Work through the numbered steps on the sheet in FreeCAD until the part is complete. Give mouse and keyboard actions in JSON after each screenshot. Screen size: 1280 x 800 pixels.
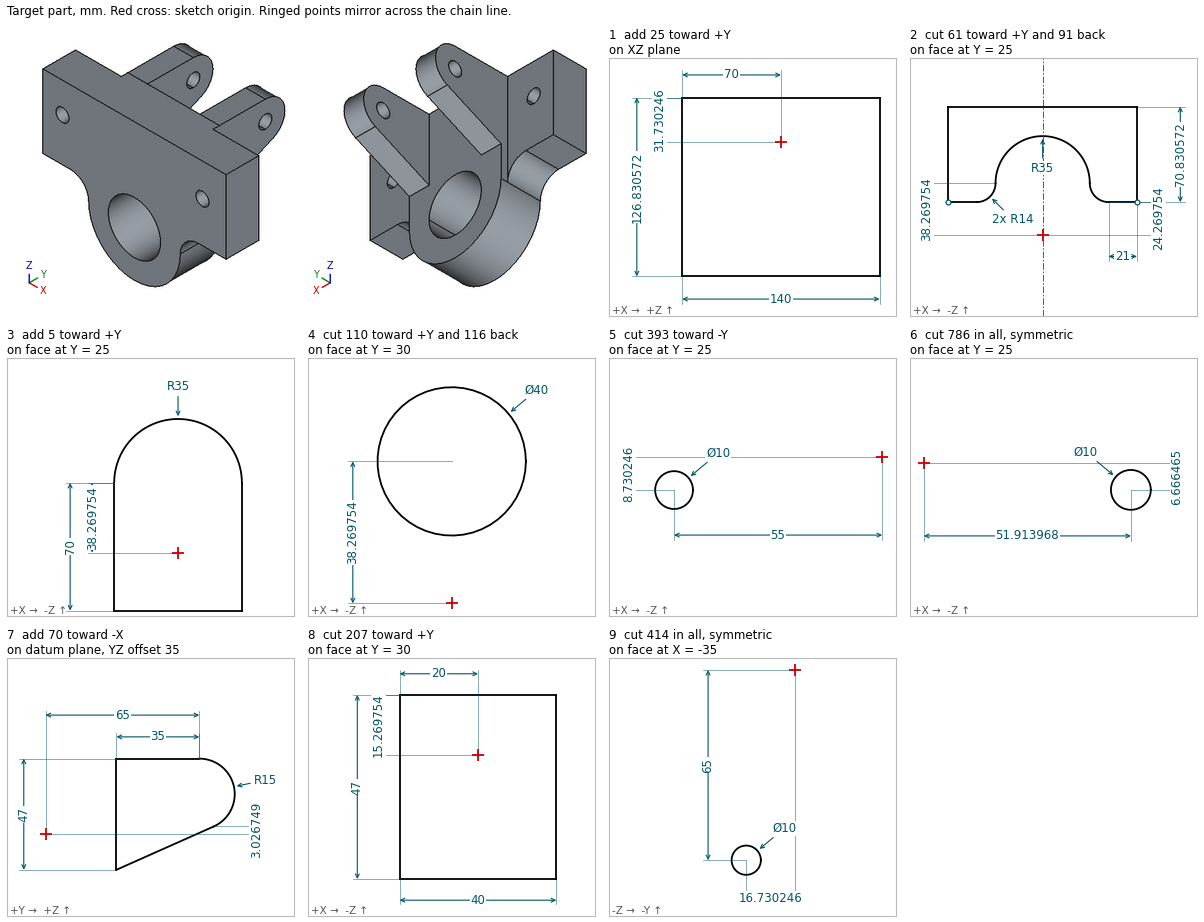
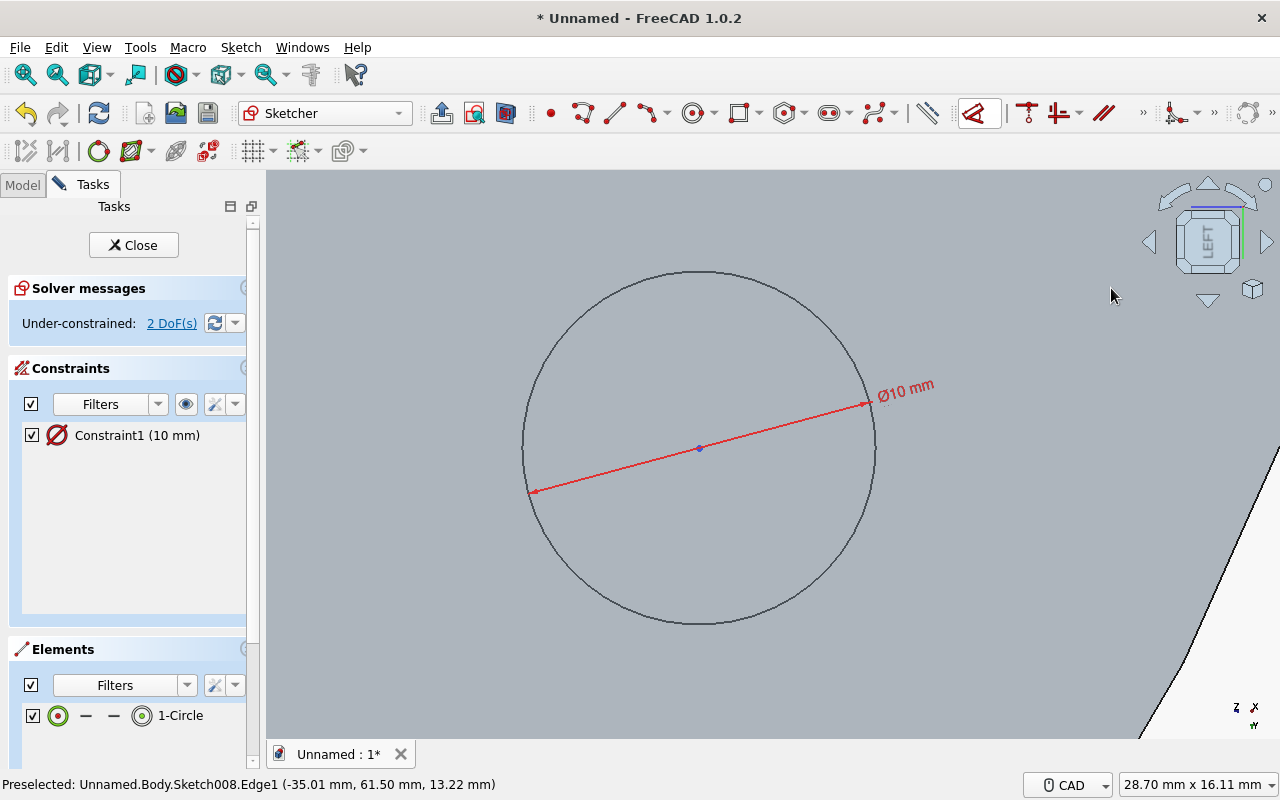
{"action": "left_click", "coordinate": [699, 448]}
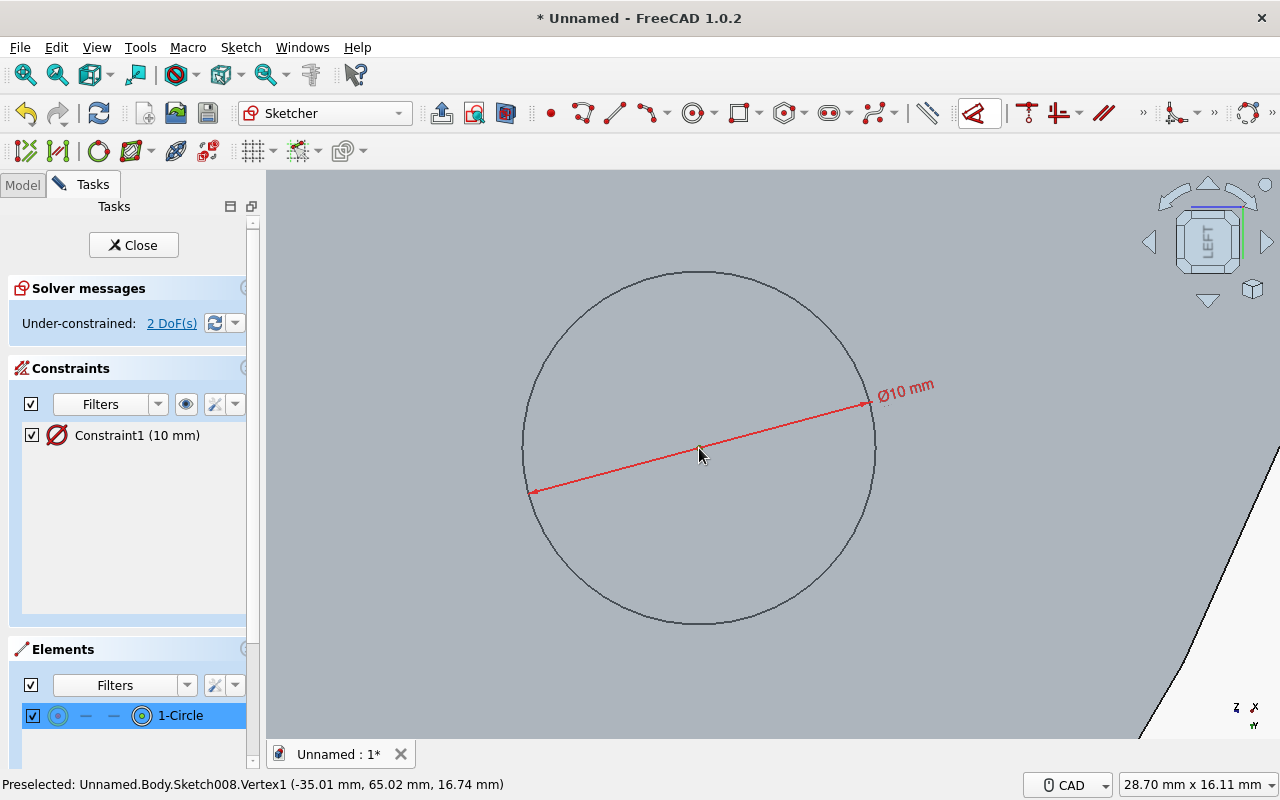
{"action": "key", "text": "i"}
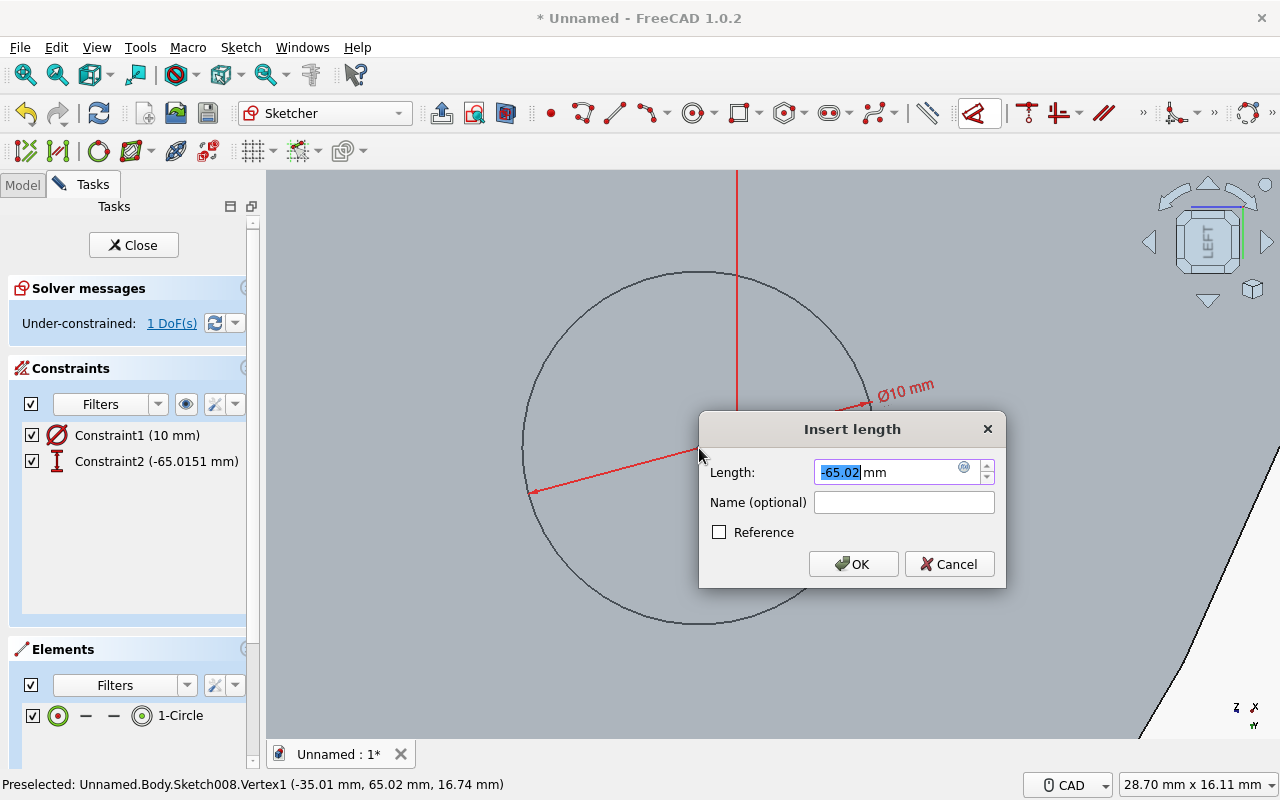
{"action": "type", "text": "-65"}
{"action": "key", "text": "Return"}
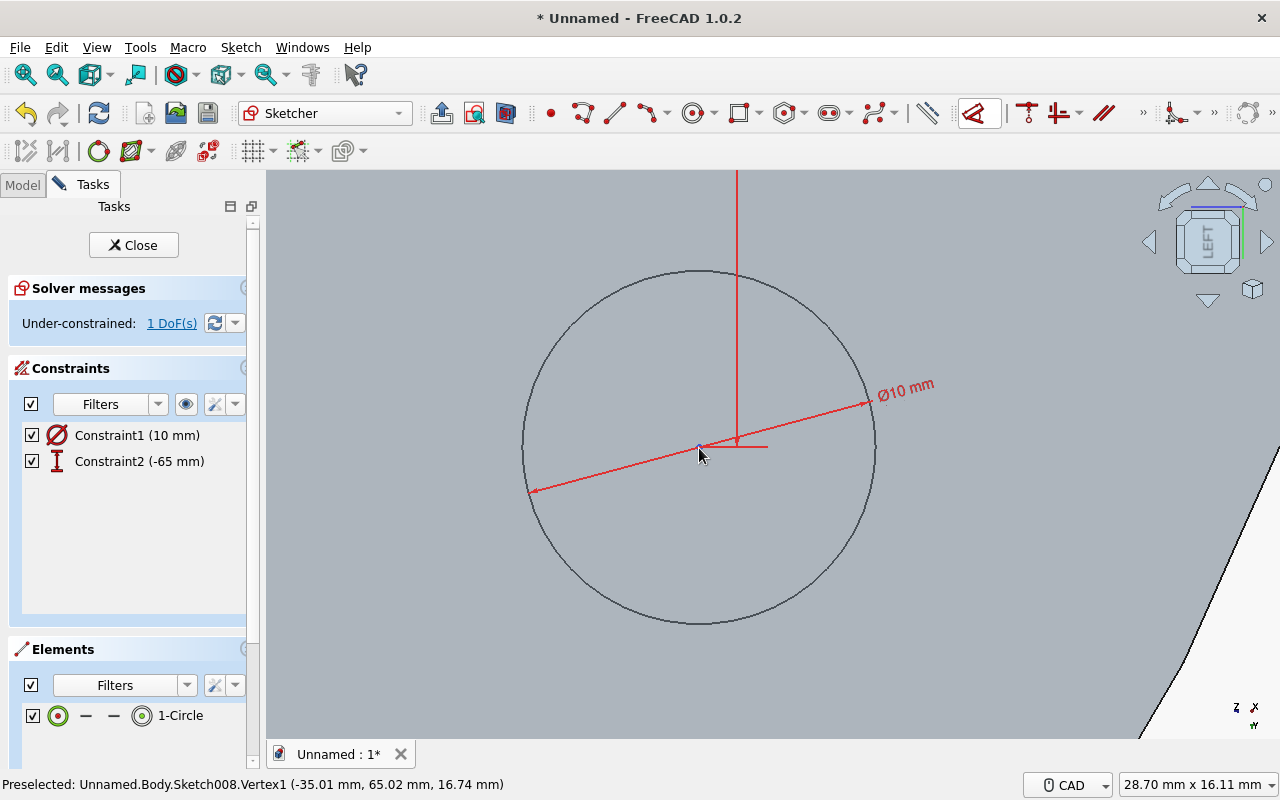
{"action": "left_click", "coordinate": [699, 447]}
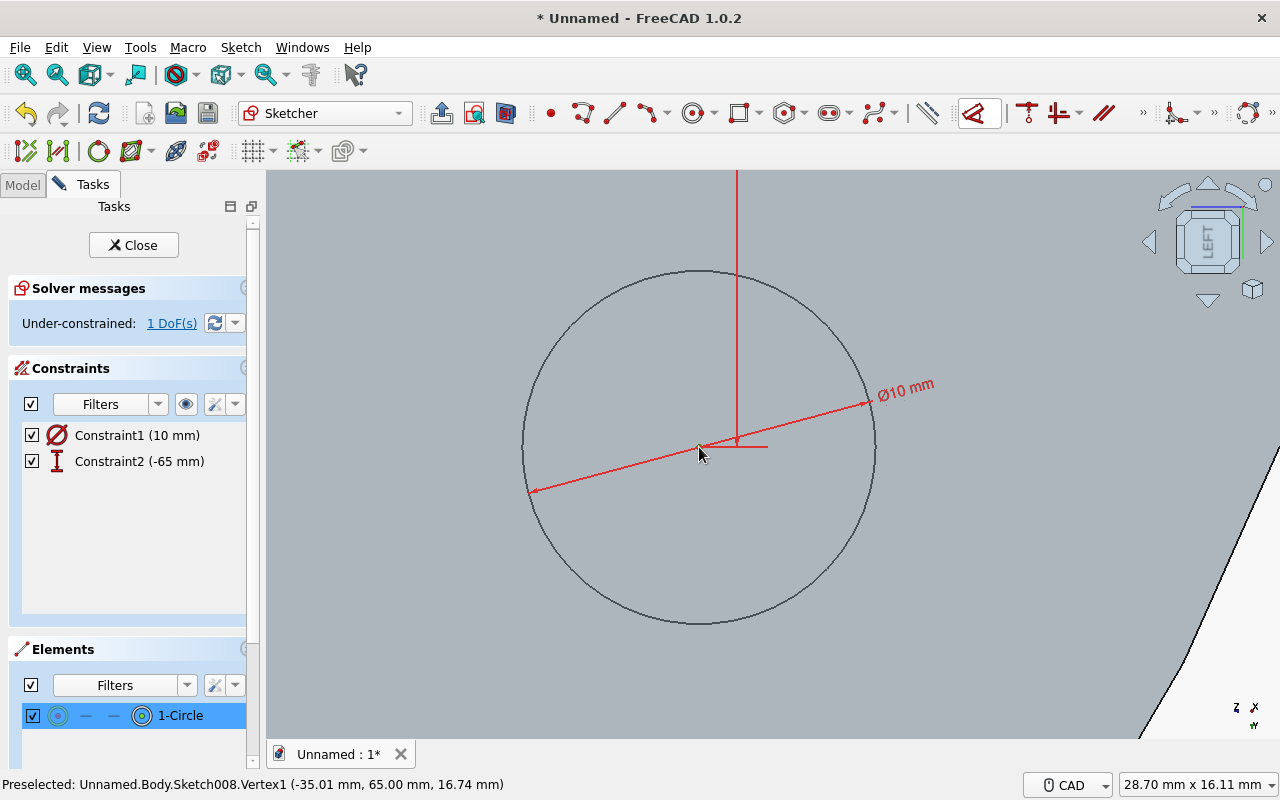
{"action": "key", "text": "l"}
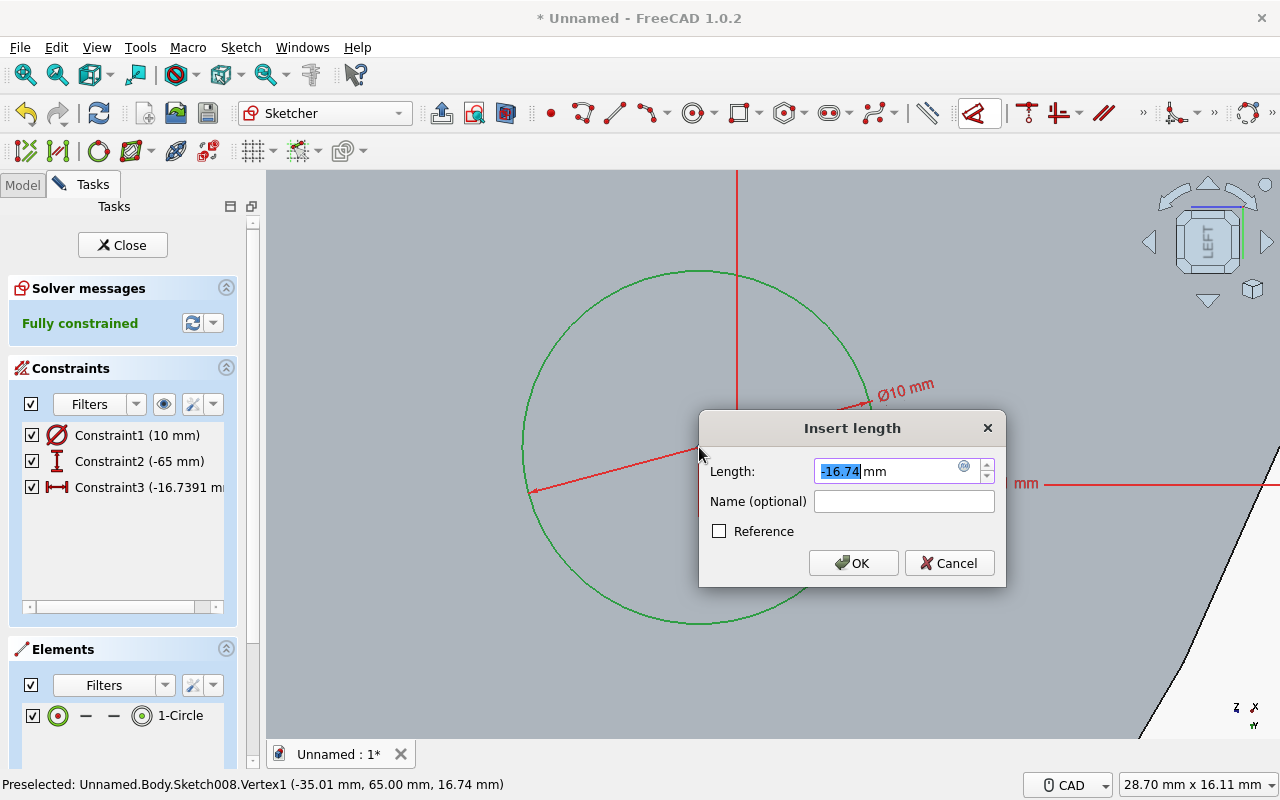
{"action": "type", "text": "-16.730246"}
{"action": "key", "text": "Return"}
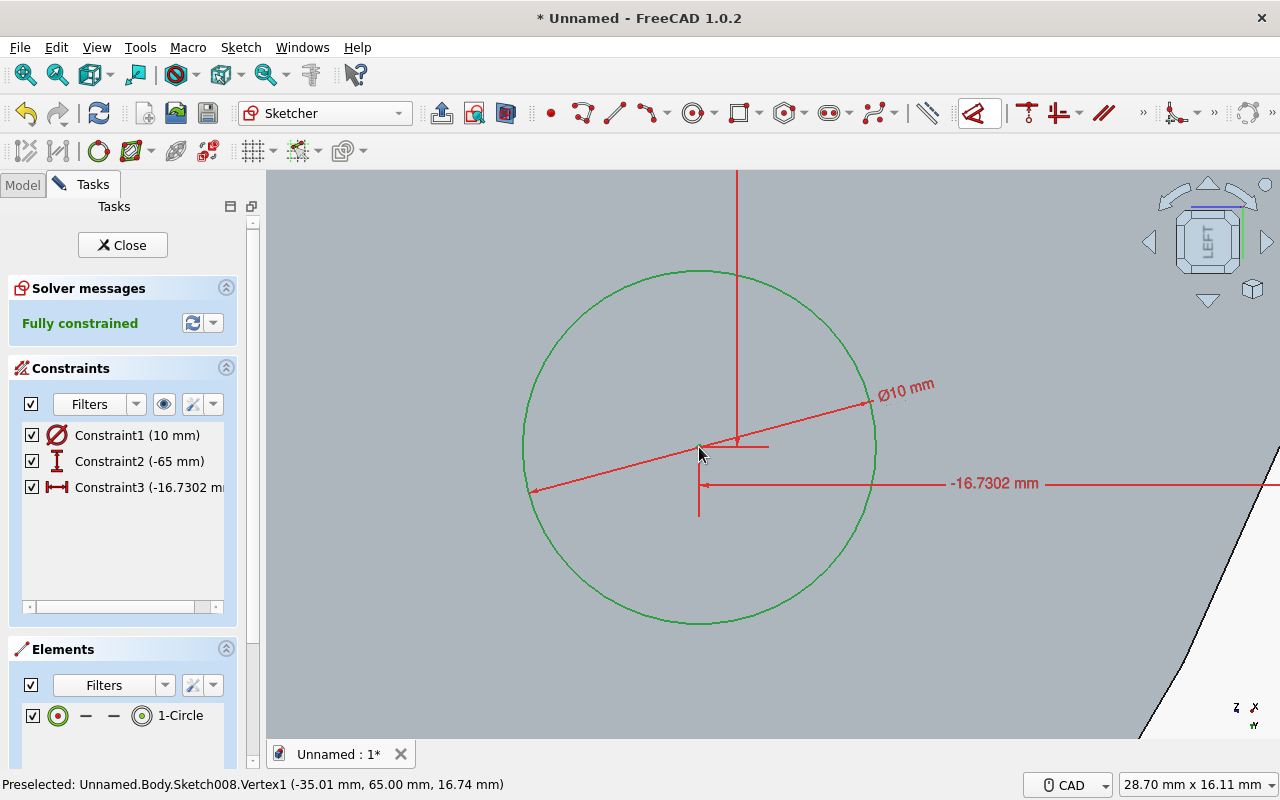
{"action": "left_click", "coordinate": [123, 245]}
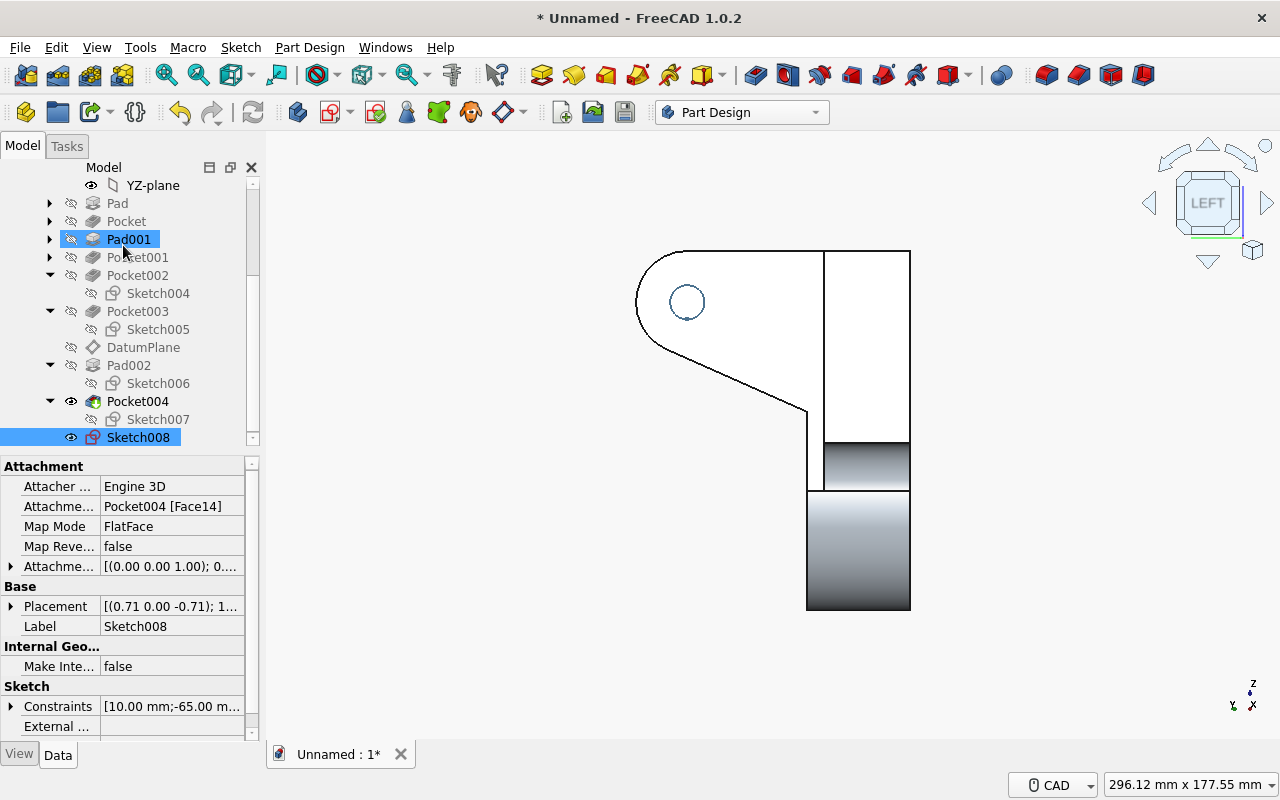
{"action": "left_click", "coordinate": [756, 76]}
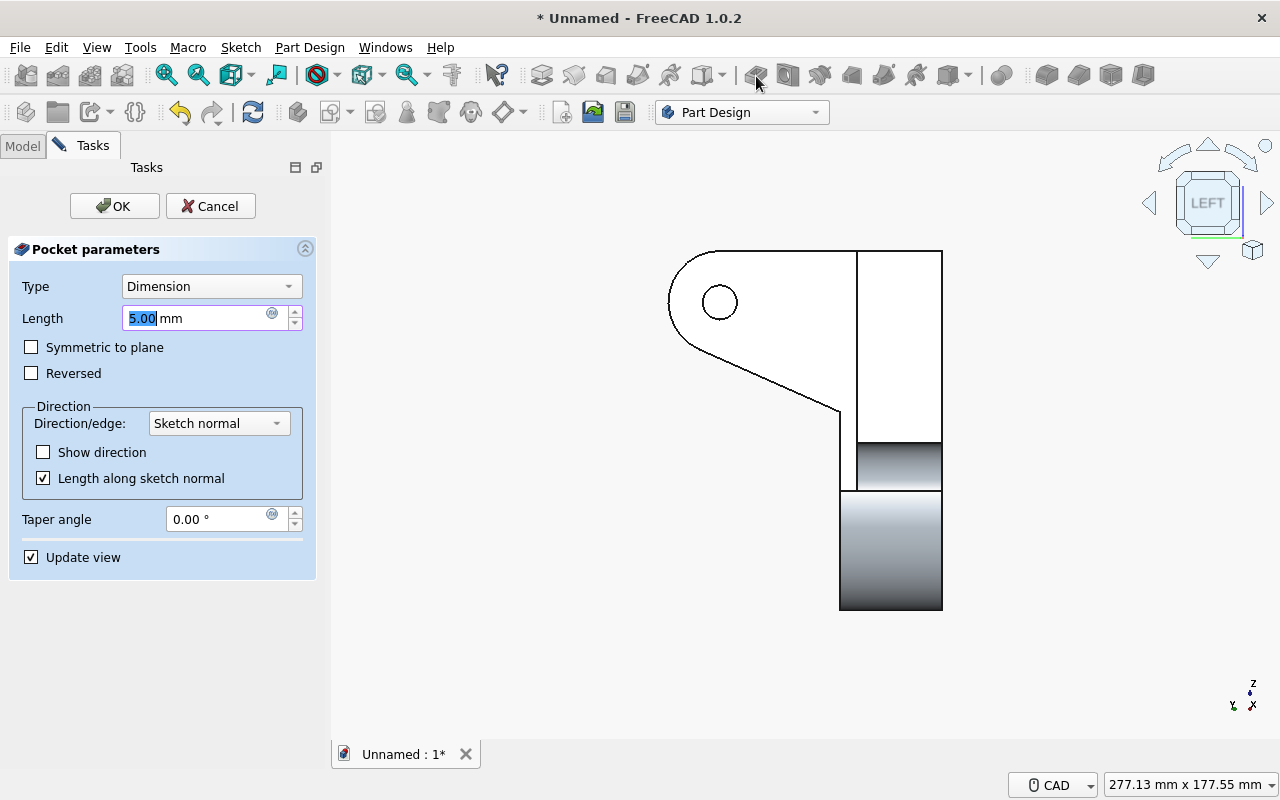
{"action": "type", "text": "414"}
{"action": "key", "text": "Tab"}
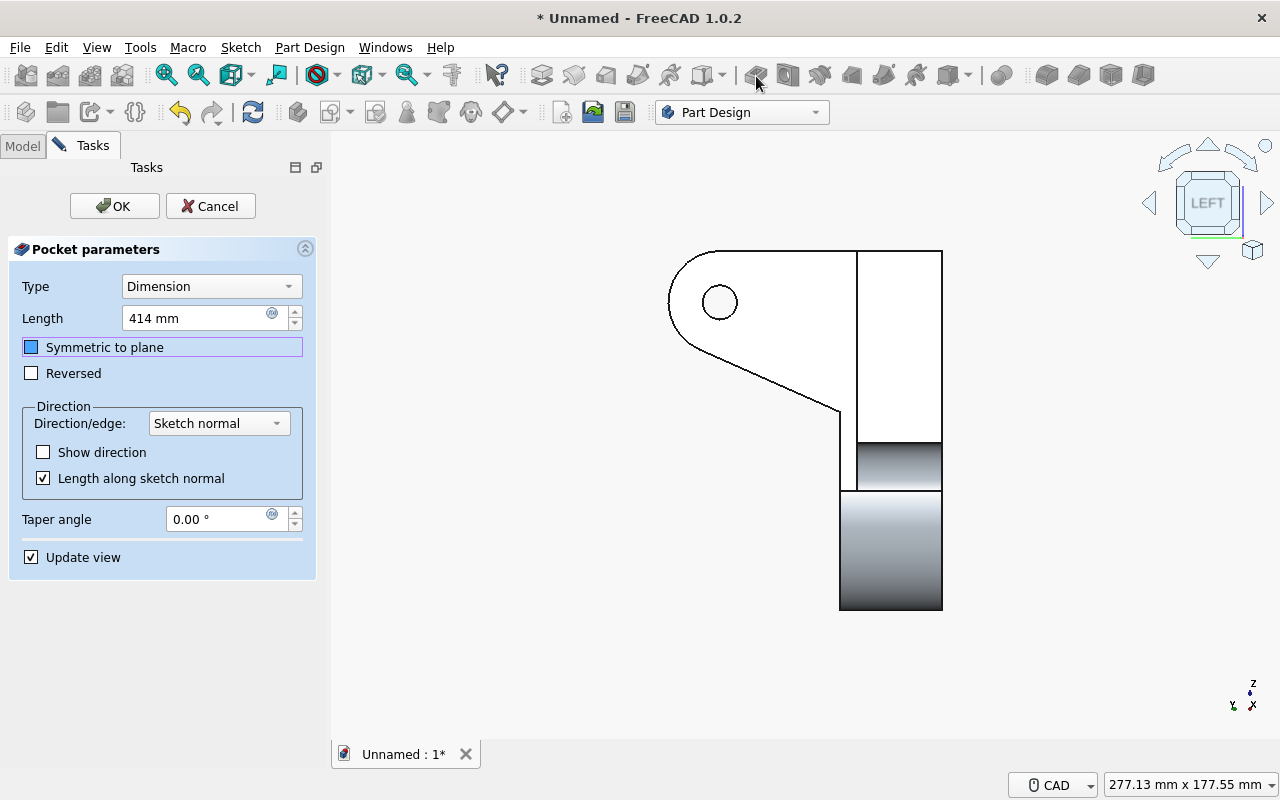
{"action": "left_click", "coordinate": [30, 347]}